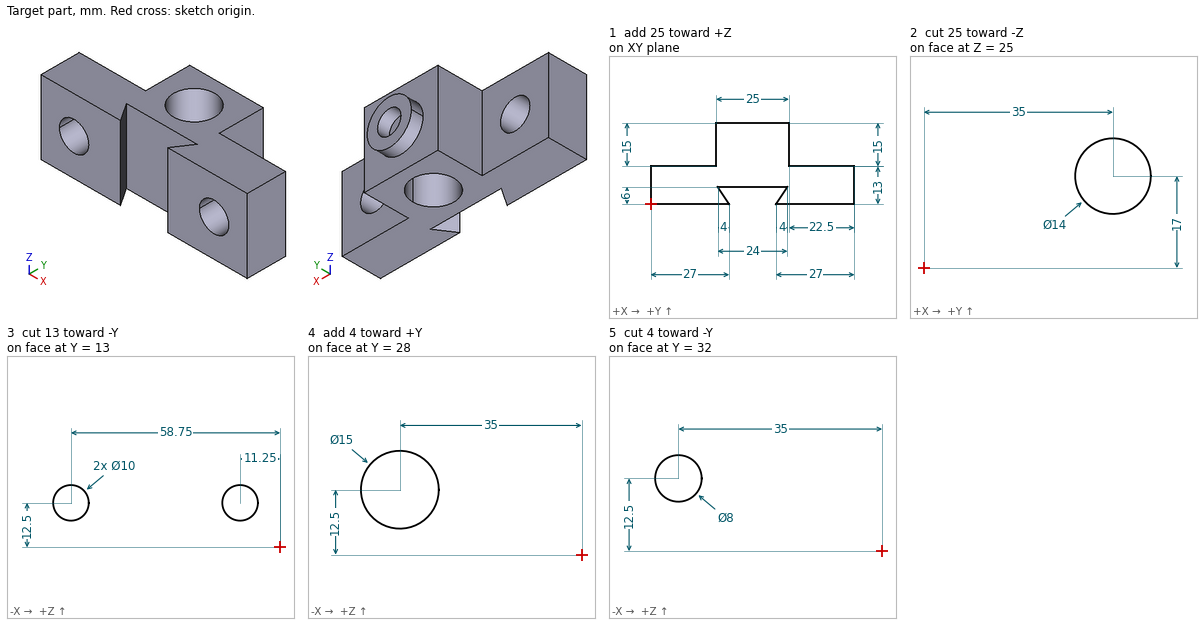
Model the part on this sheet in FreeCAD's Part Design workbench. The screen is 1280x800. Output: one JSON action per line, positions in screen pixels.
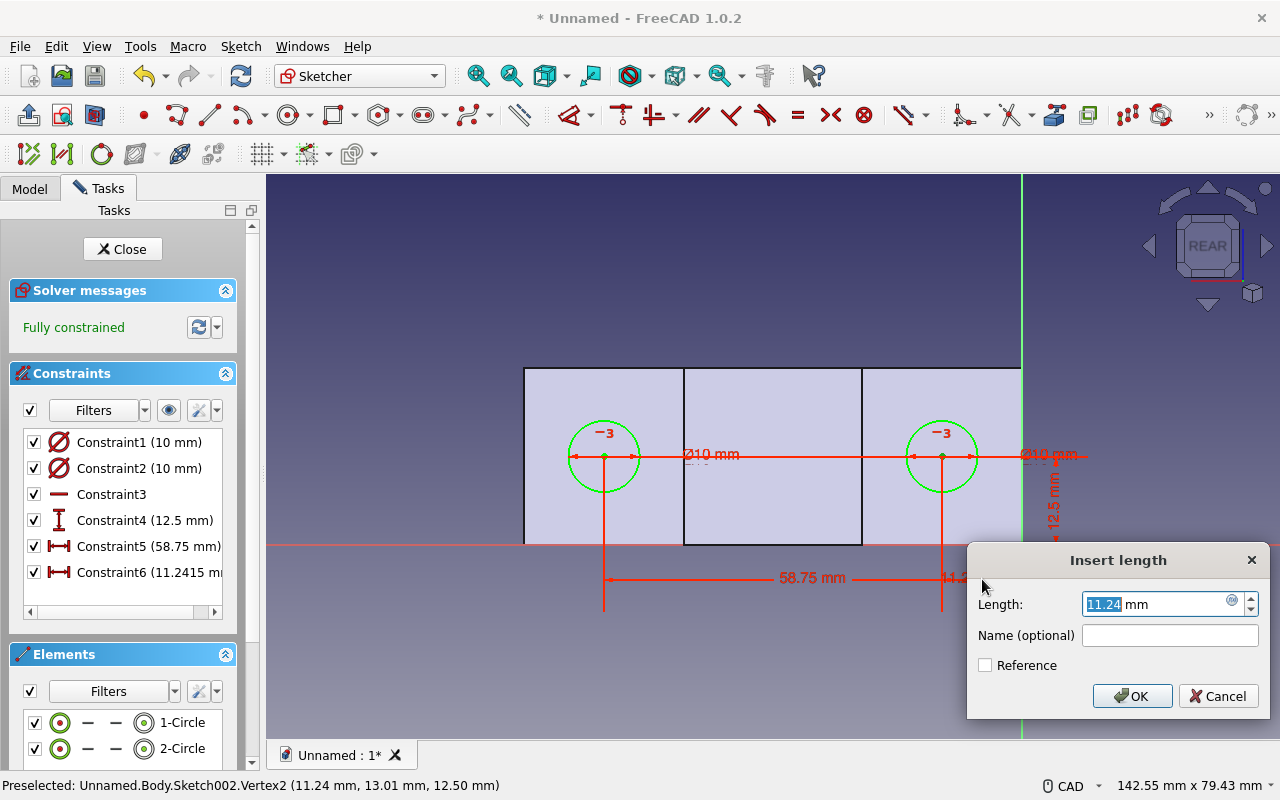
{"action": "type", "text": "11.25"}
{"action": "key", "text": "Return"}
{"action": "key", "text": "Escape"}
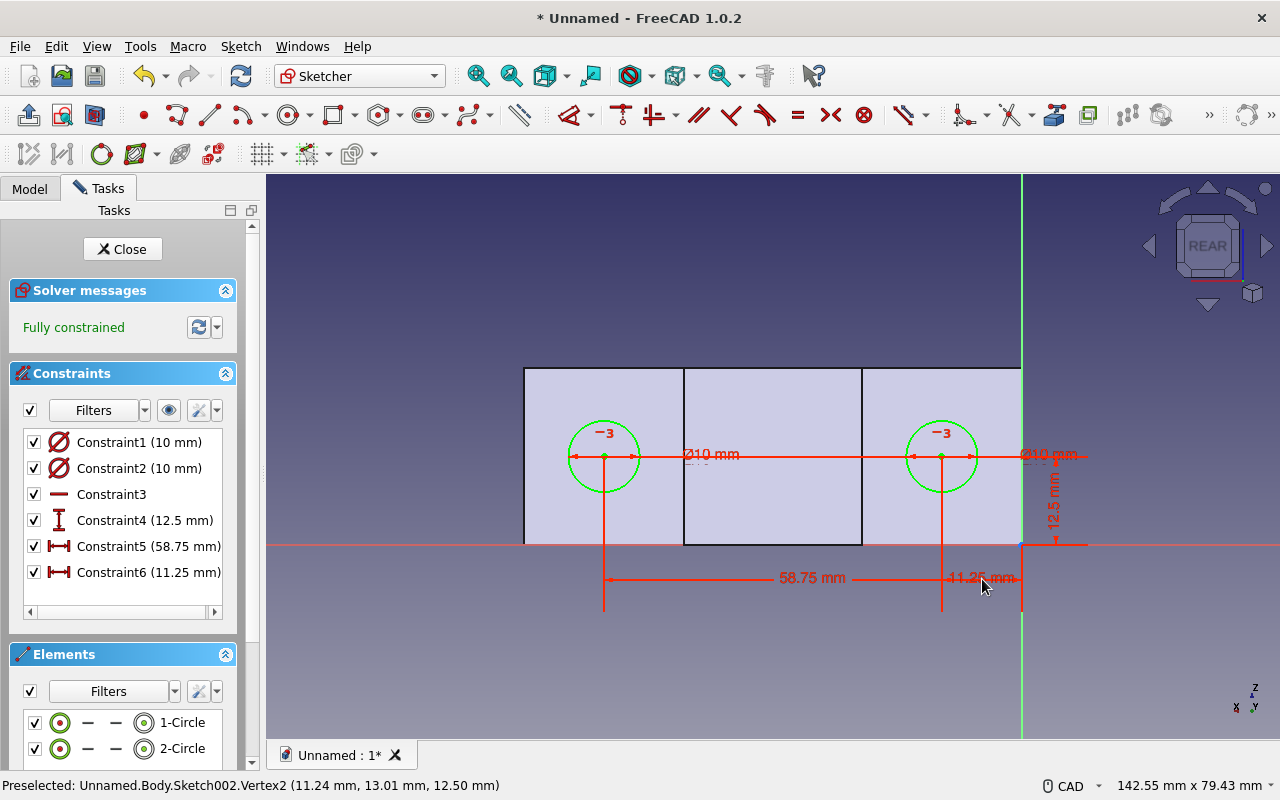
{"action": "left_click", "coordinate": [123, 249]}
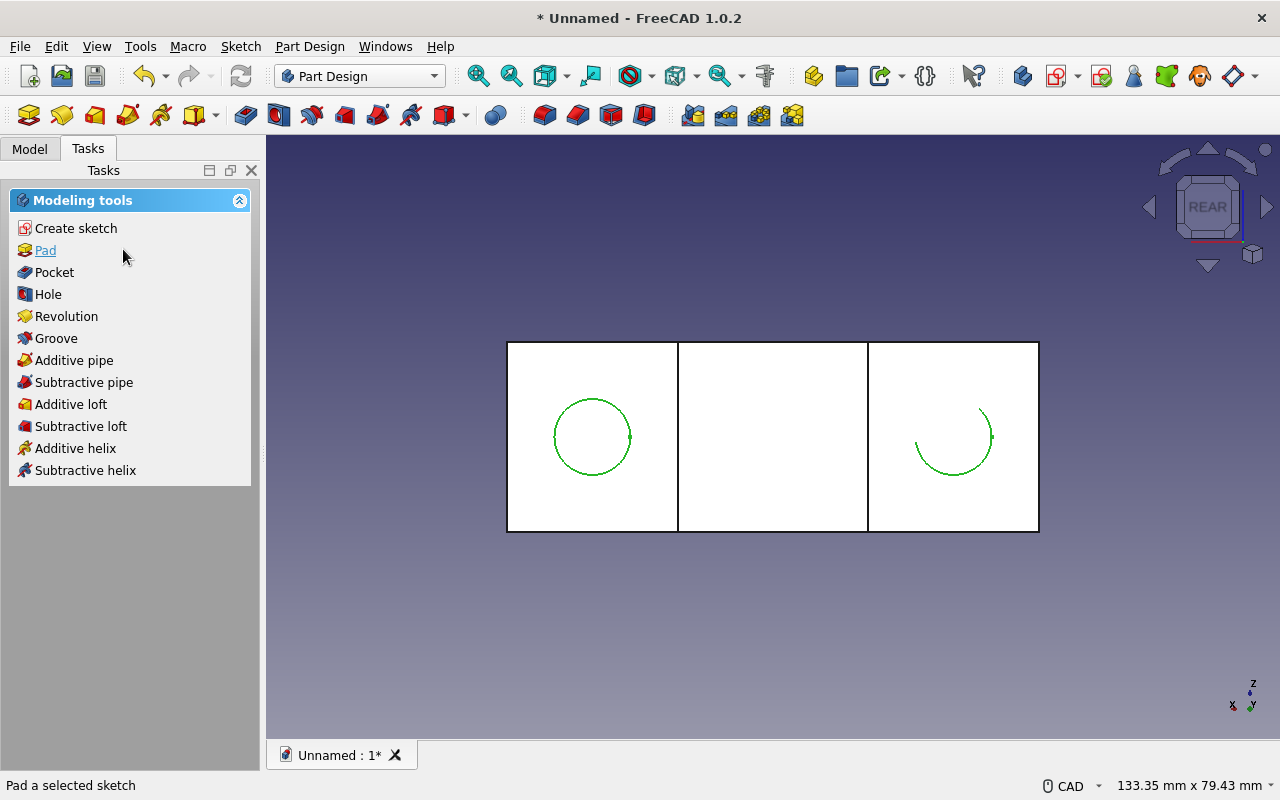
{"action": "left_click", "coordinate": [246, 116]}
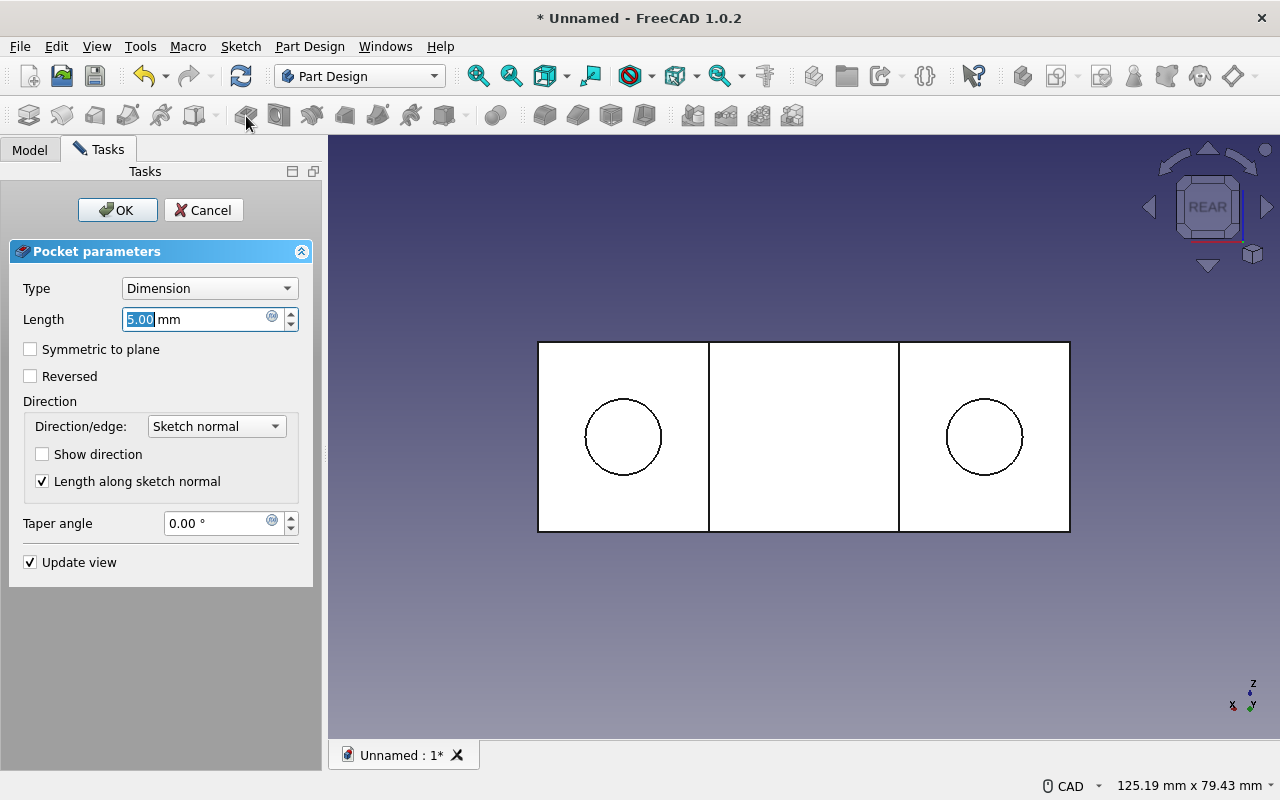
{"action": "type", "text": "13"}
{"action": "key", "text": "Tab"}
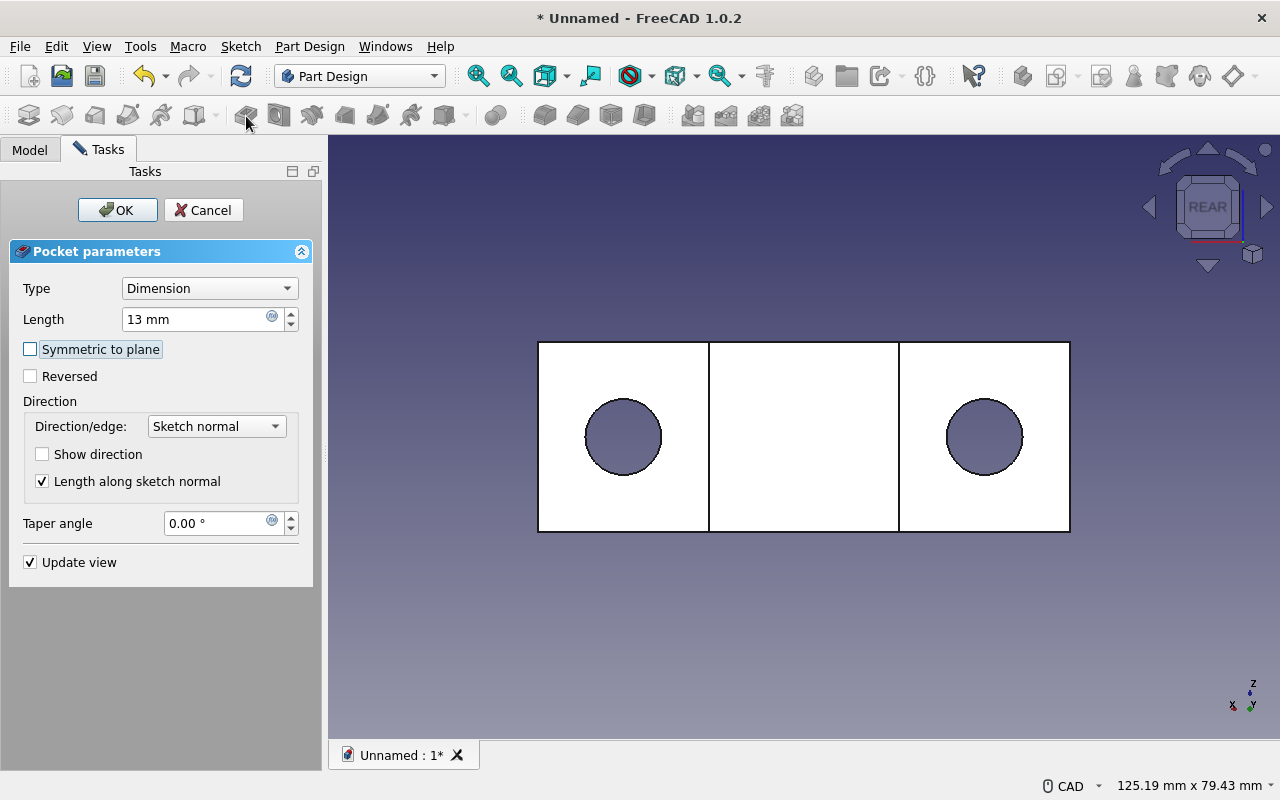
{"action": "left_click", "coordinate": [118, 210]}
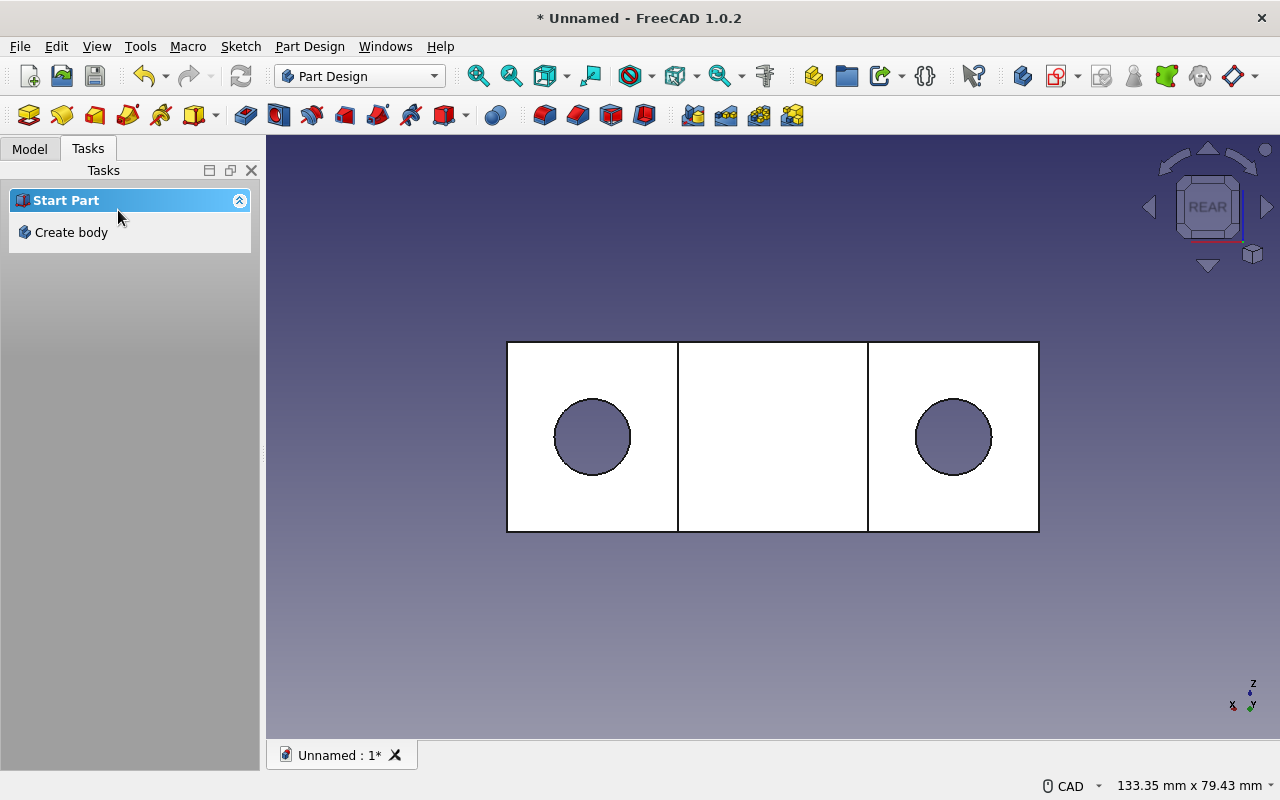
{"action": "left_click", "coordinate": [773, 436]}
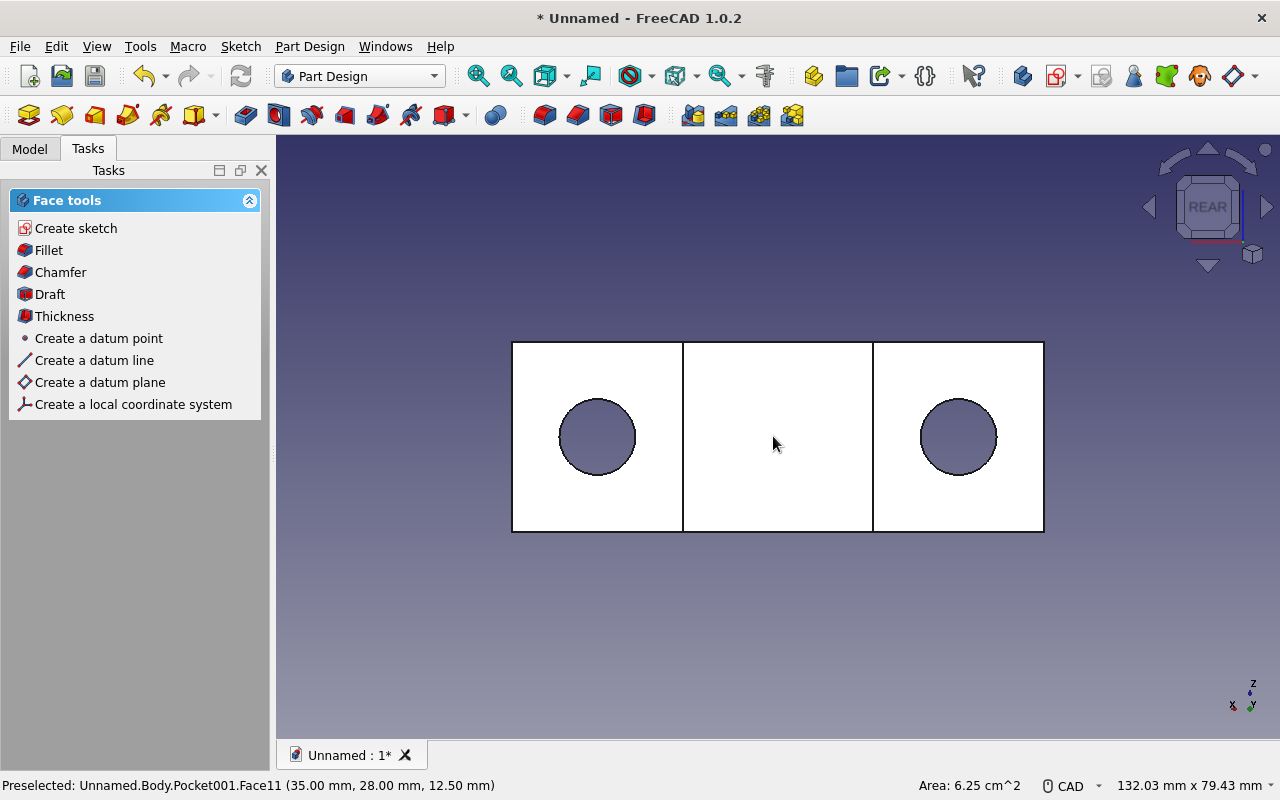
{"action": "left_click", "coordinate": [1056, 76]}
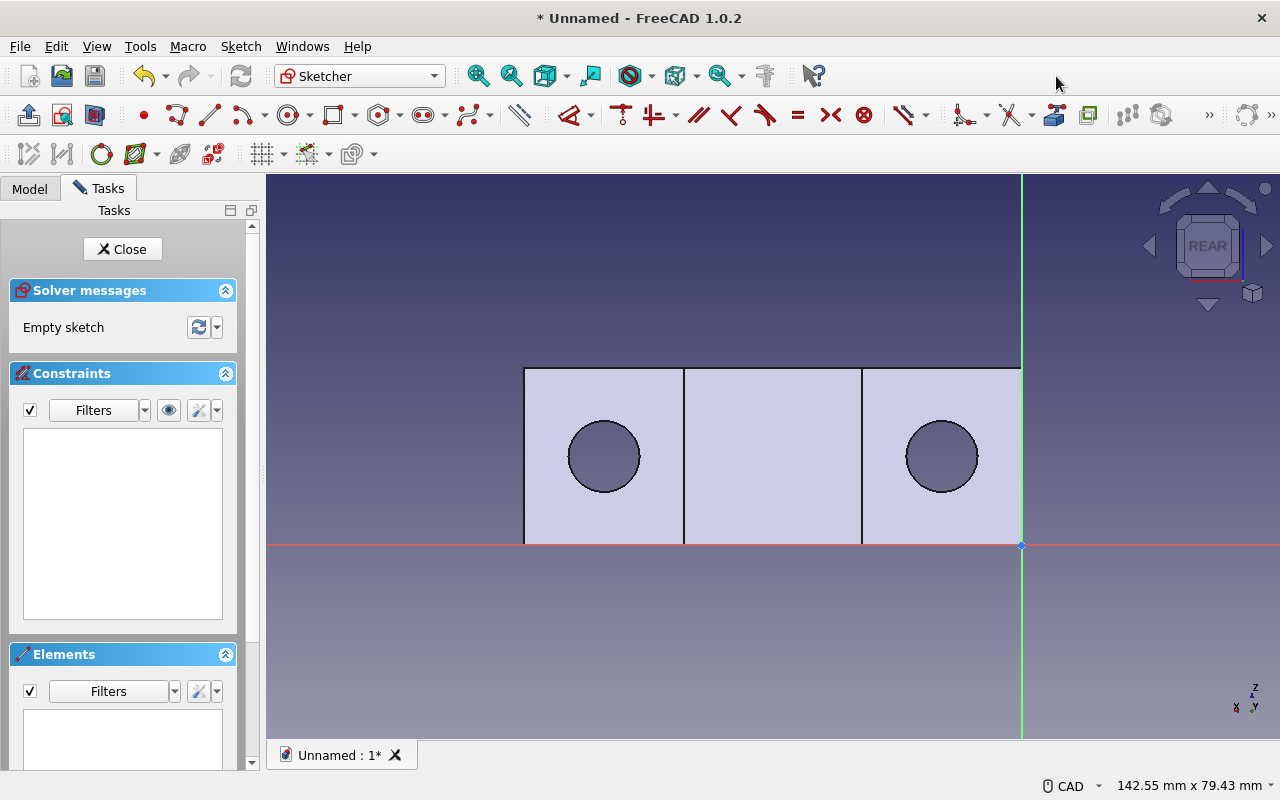
{"action": "scroll", "coordinate": [803, 457], "scroll_direction": "up", "scroll_amount": 6}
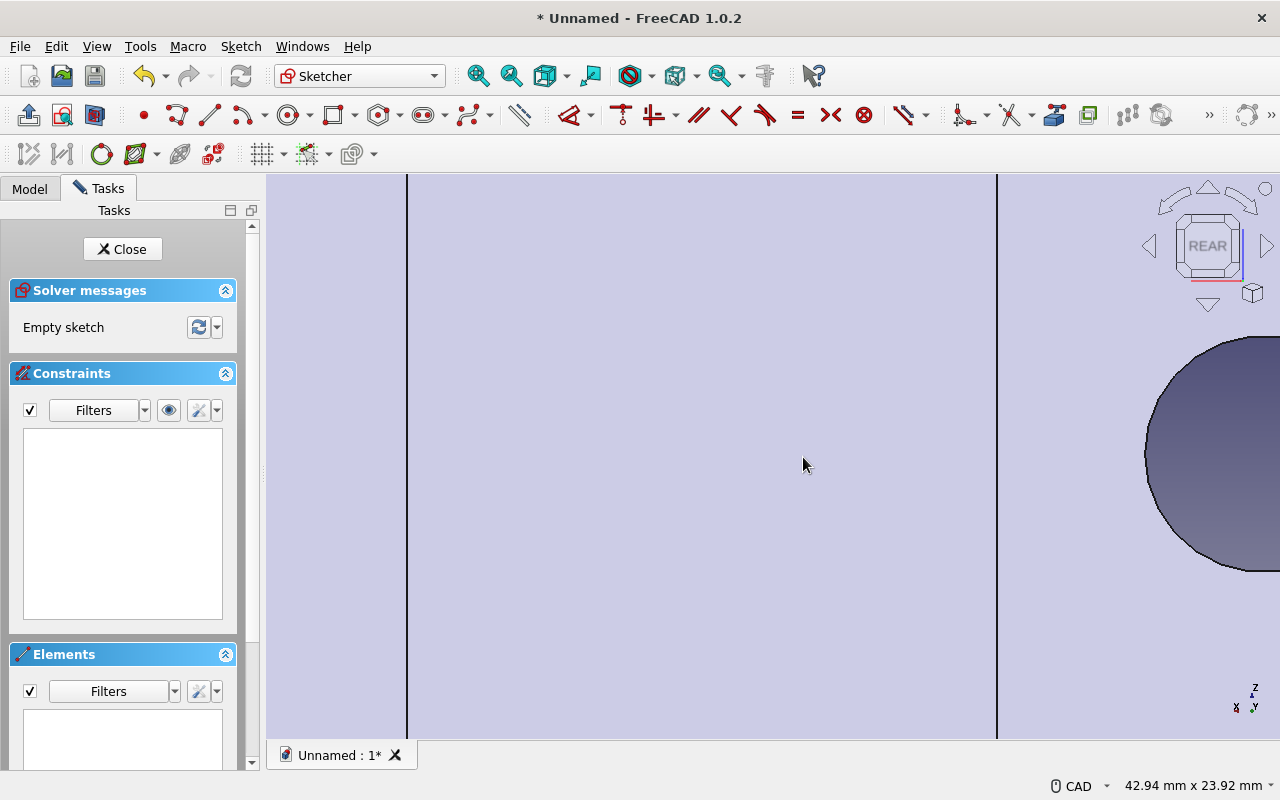
{"action": "left_click", "coordinate": [288, 116]}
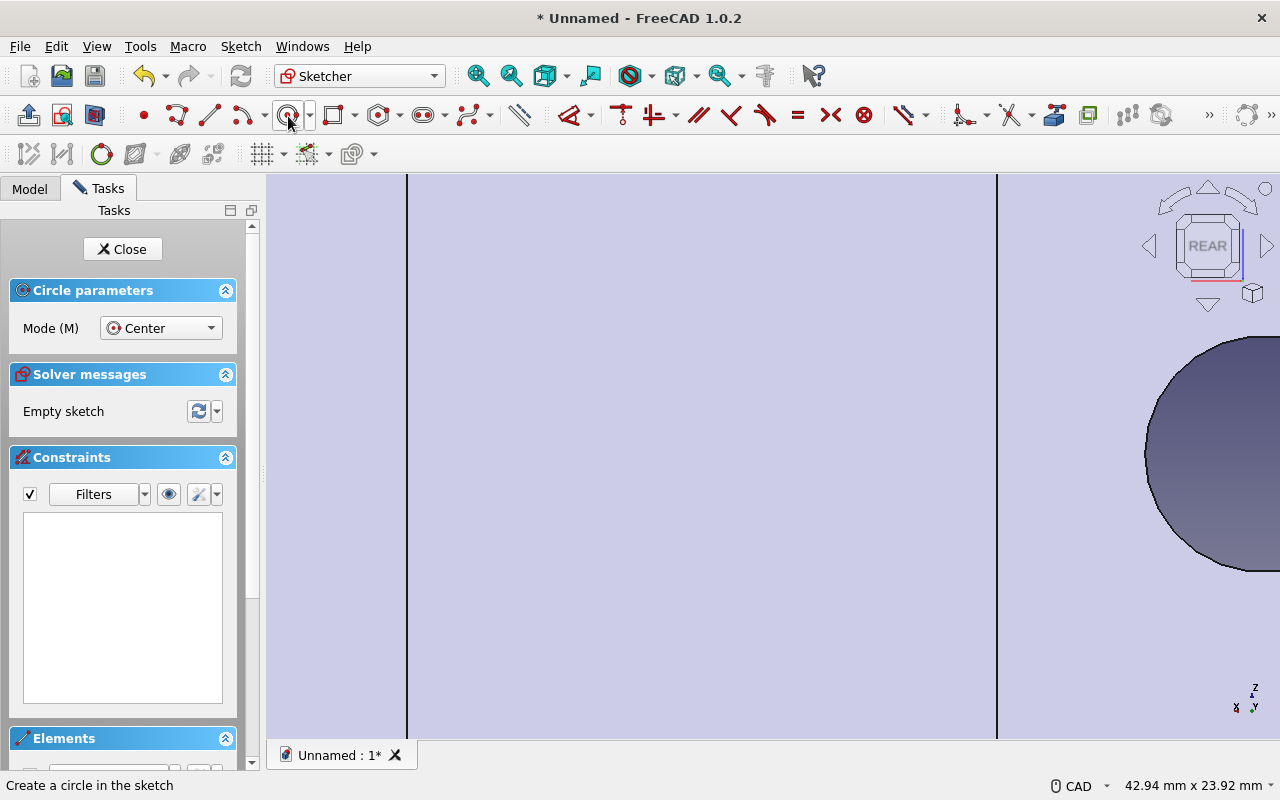
{"action": "left_click", "coordinate": [702, 454]}
{"action": "mouse_move", "coordinate": [827, 329]}